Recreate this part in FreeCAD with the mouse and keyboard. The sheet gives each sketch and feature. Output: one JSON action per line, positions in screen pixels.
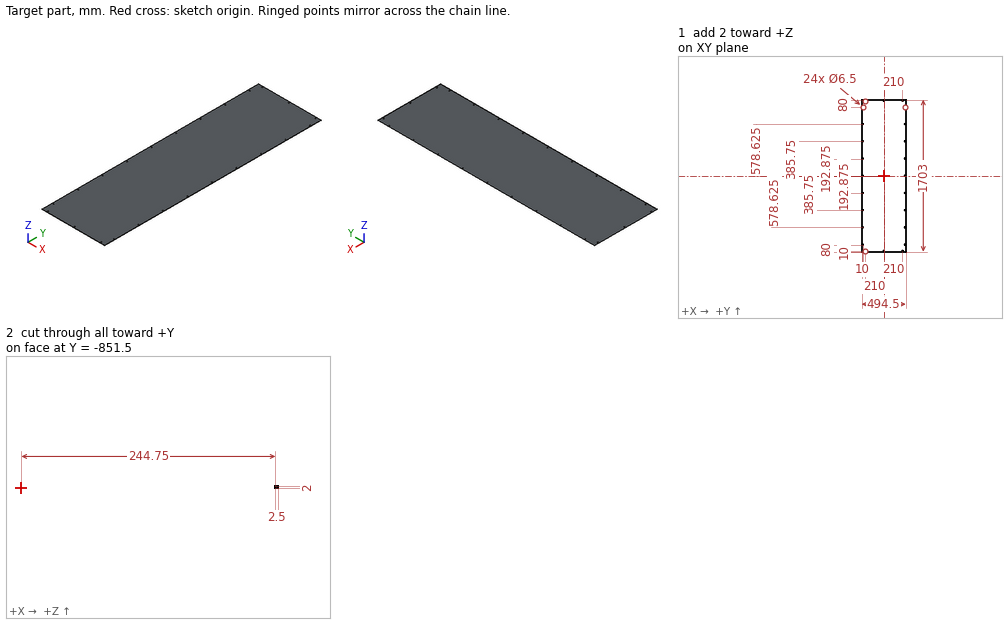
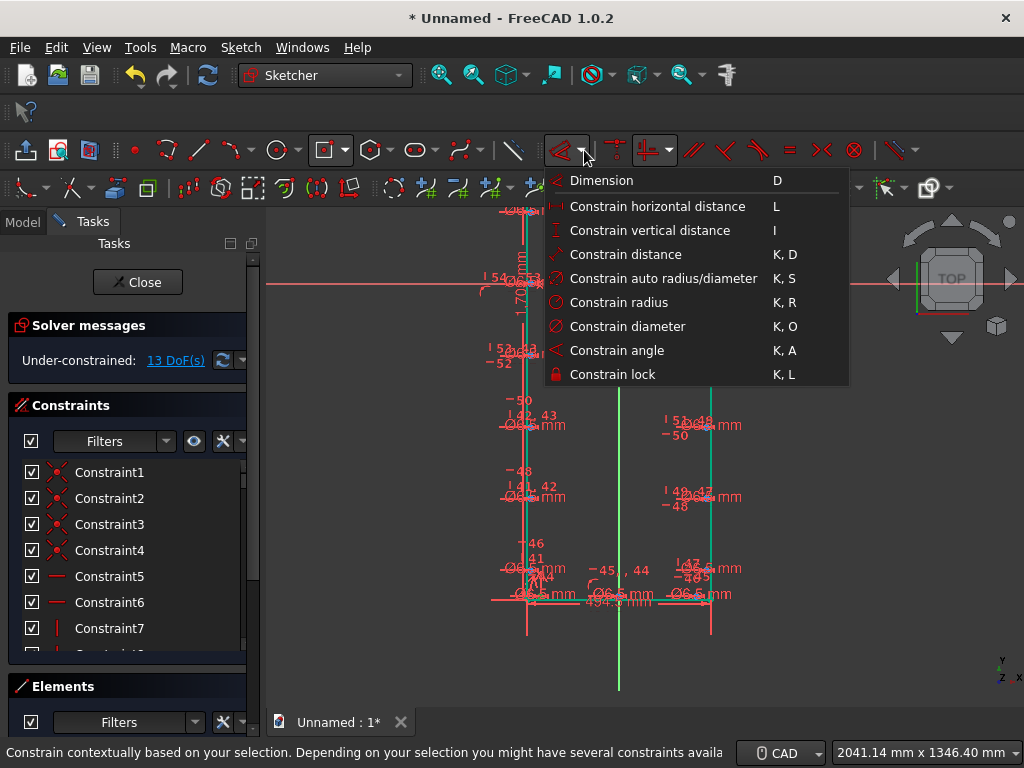
{"action": "left_click", "coordinate": [697, 206]}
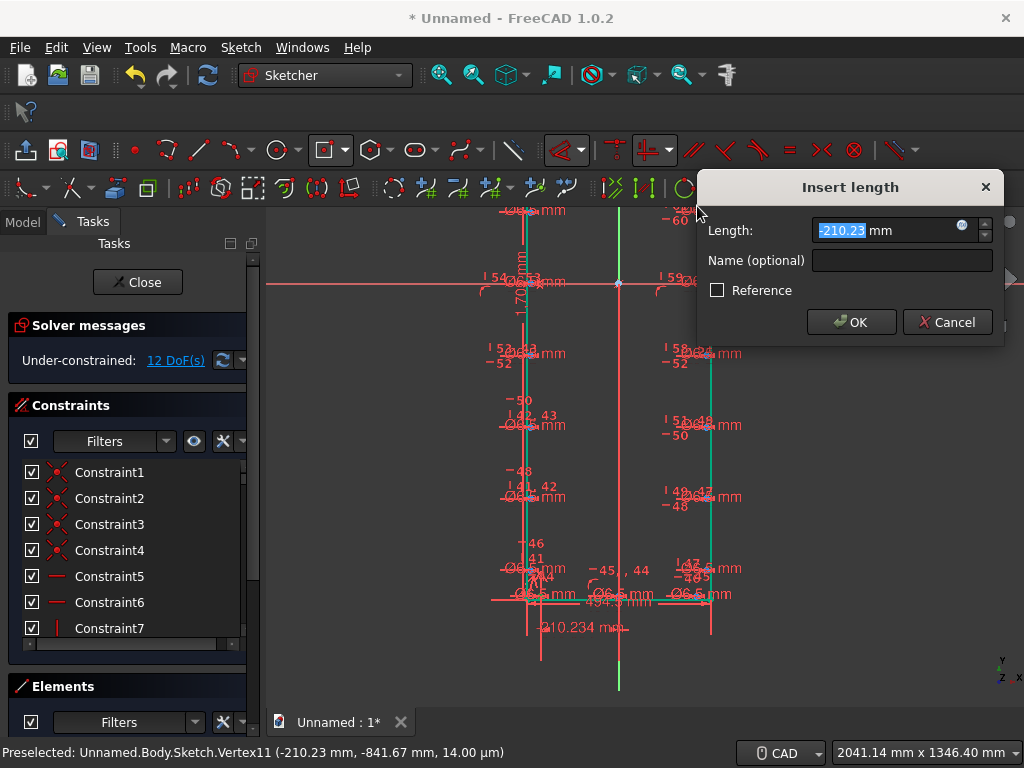
{"action": "type", "text": "-210"}
{"action": "key", "text": "Return"}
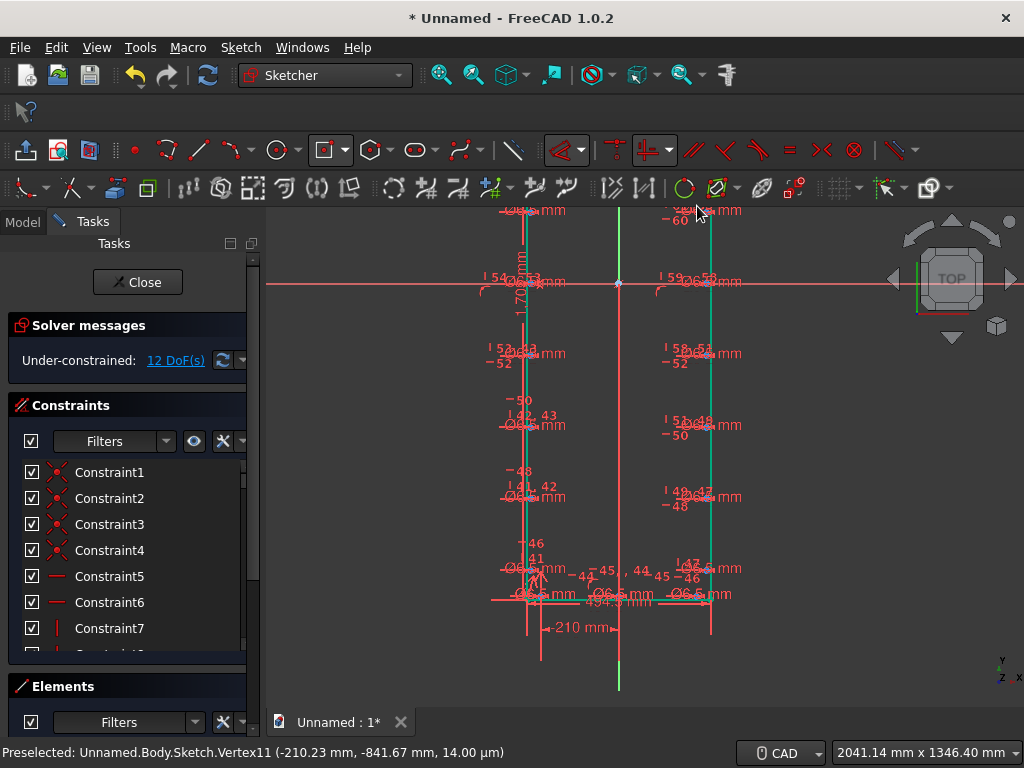
{"action": "left_click", "coordinate": [697, 596]}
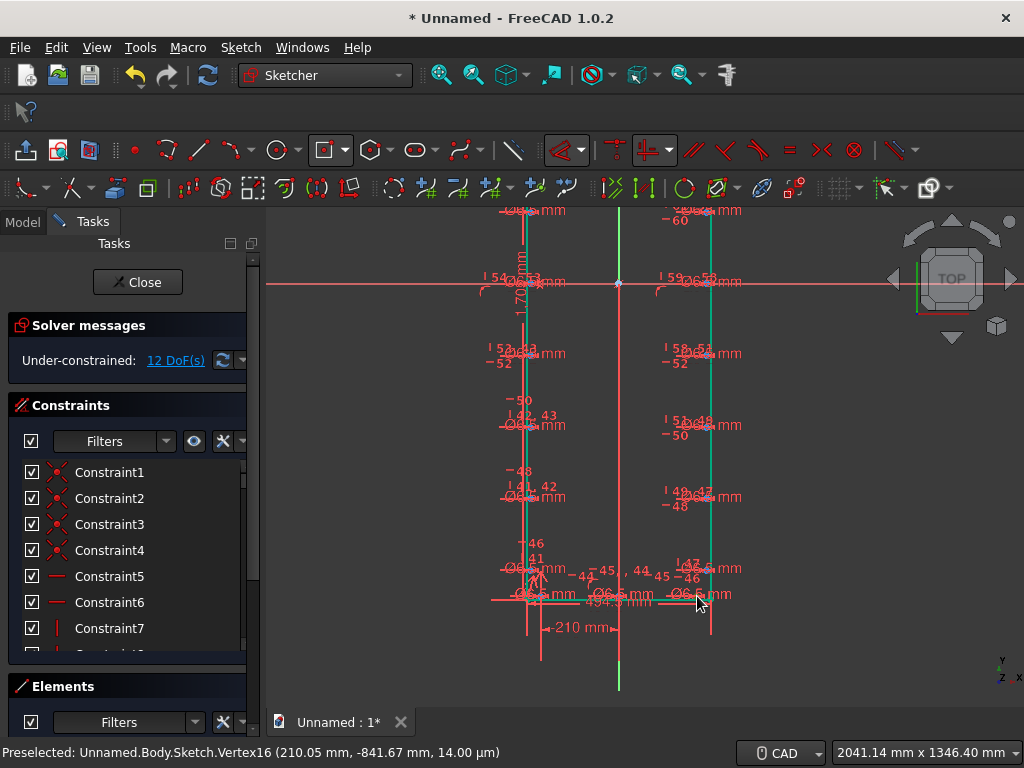
{"action": "left_click", "coordinate": [584, 150]}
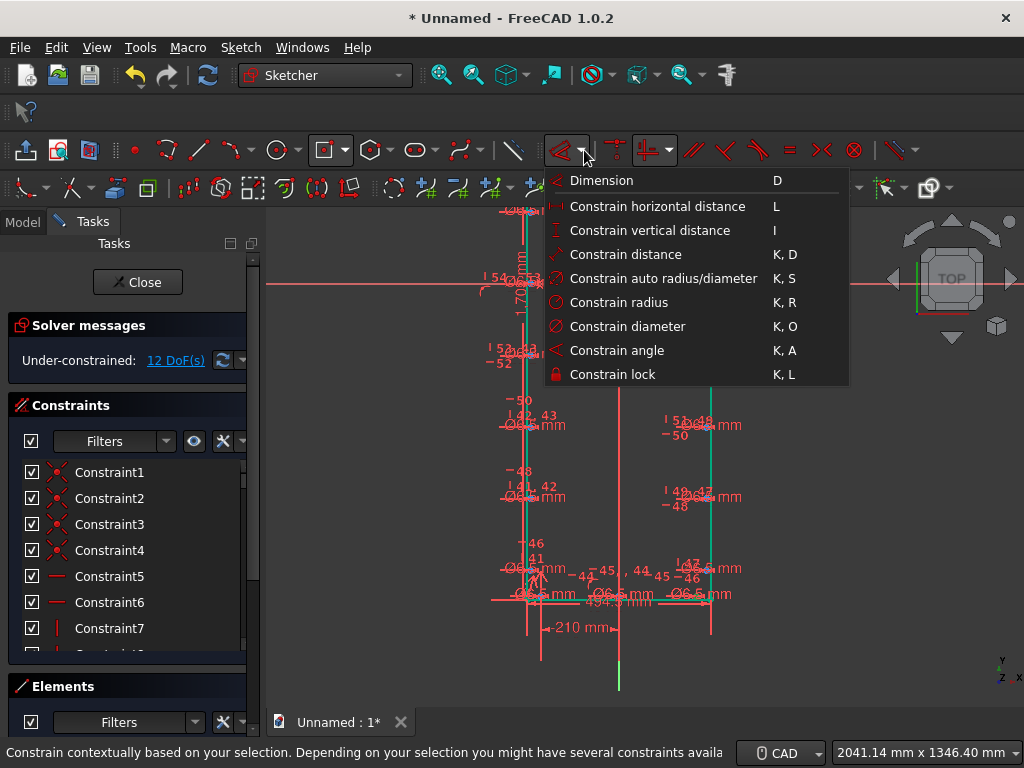
{"action": "left_click", "coordinate": [697, 206]}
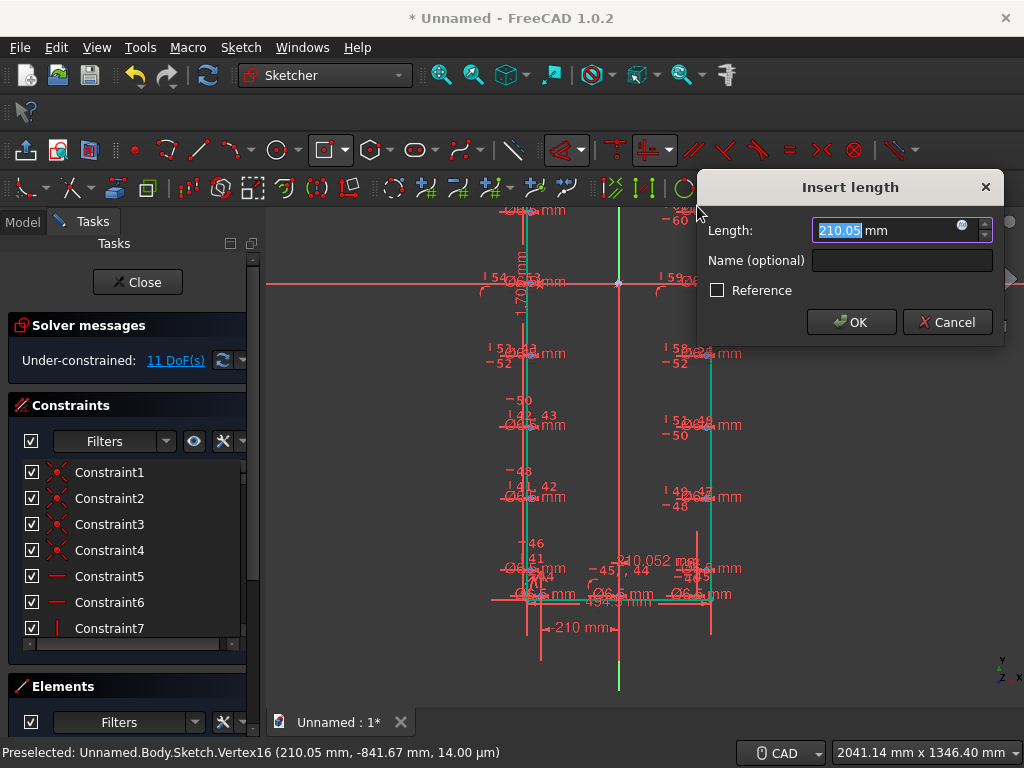
{"action": "type", "text": "210"}
{"action": "key", "text": "Return"}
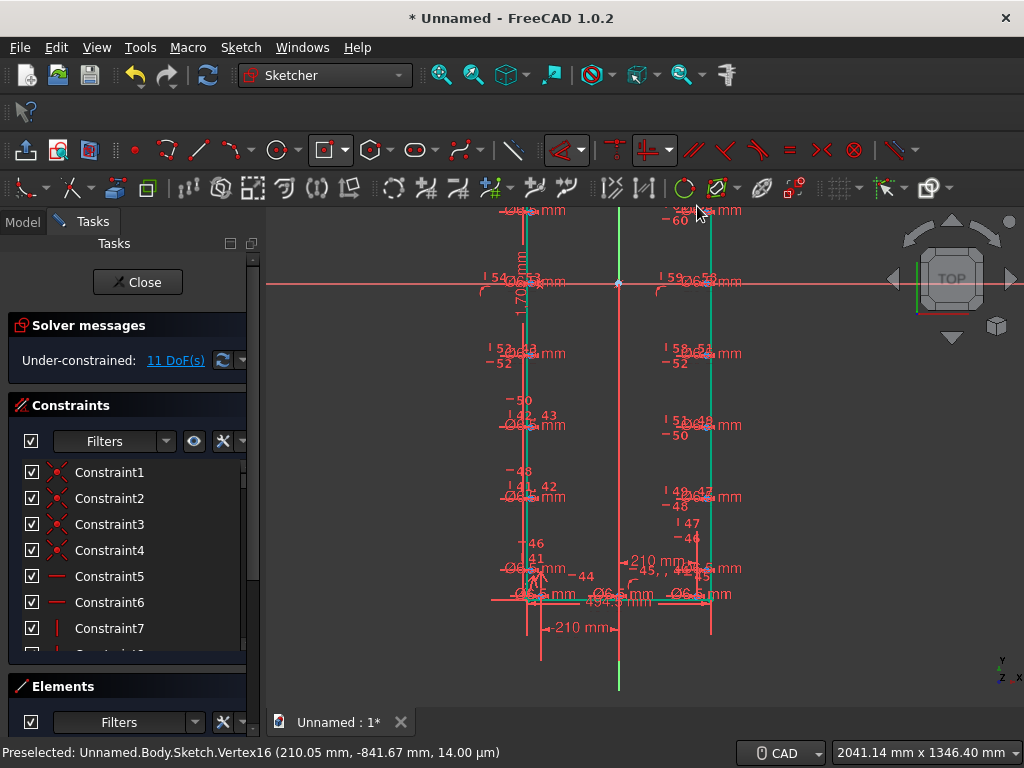
{"action": "scroll", "coordinate": [542, 598], "scroll_direction": "down", "scroll_amount": 4}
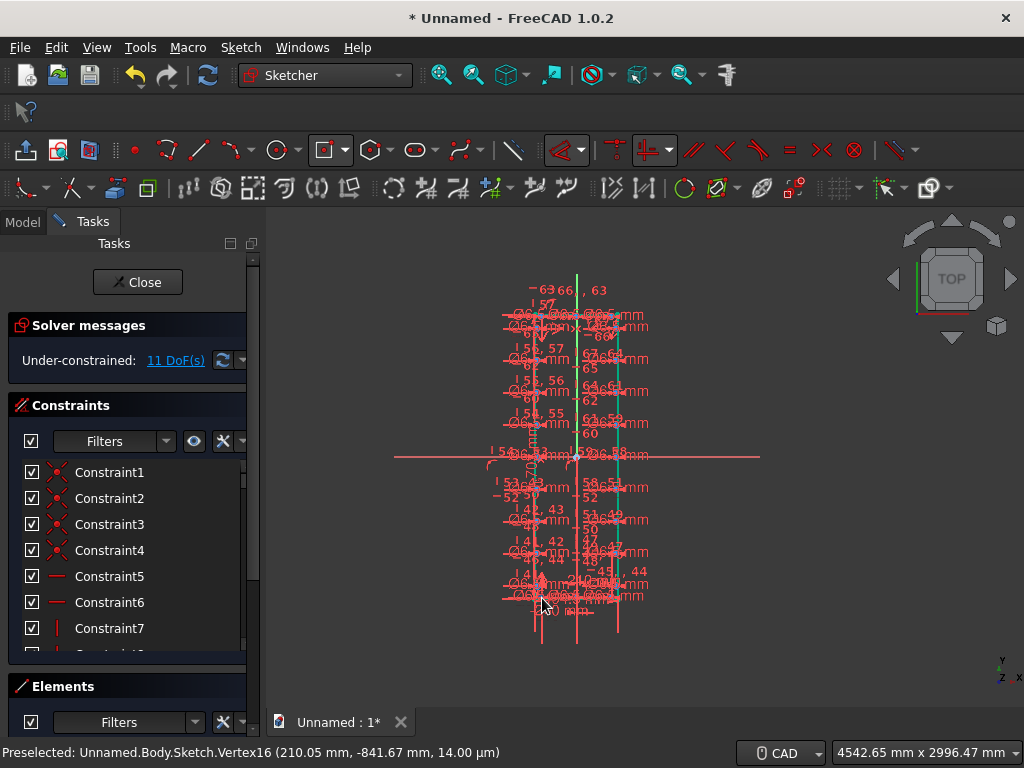
{"action": "scroll", "coordinate": [612, 317], "scroll_direction": "up", "scroll_amount": 4}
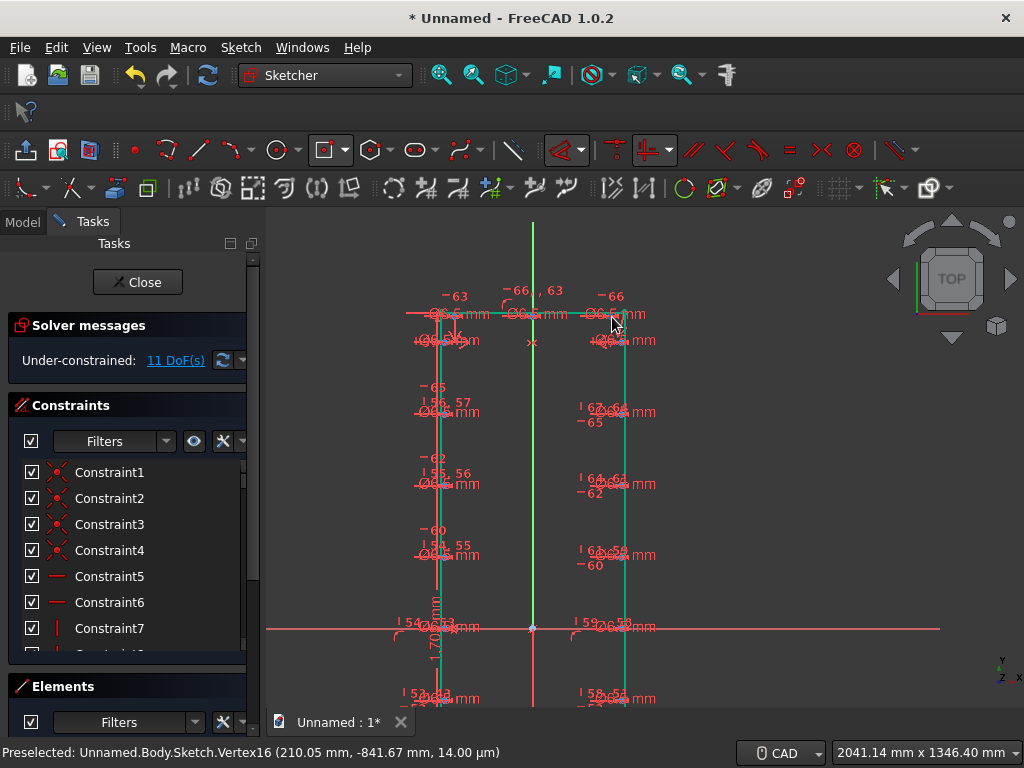
{"action": "left_click", "coordinate": [611, 316]}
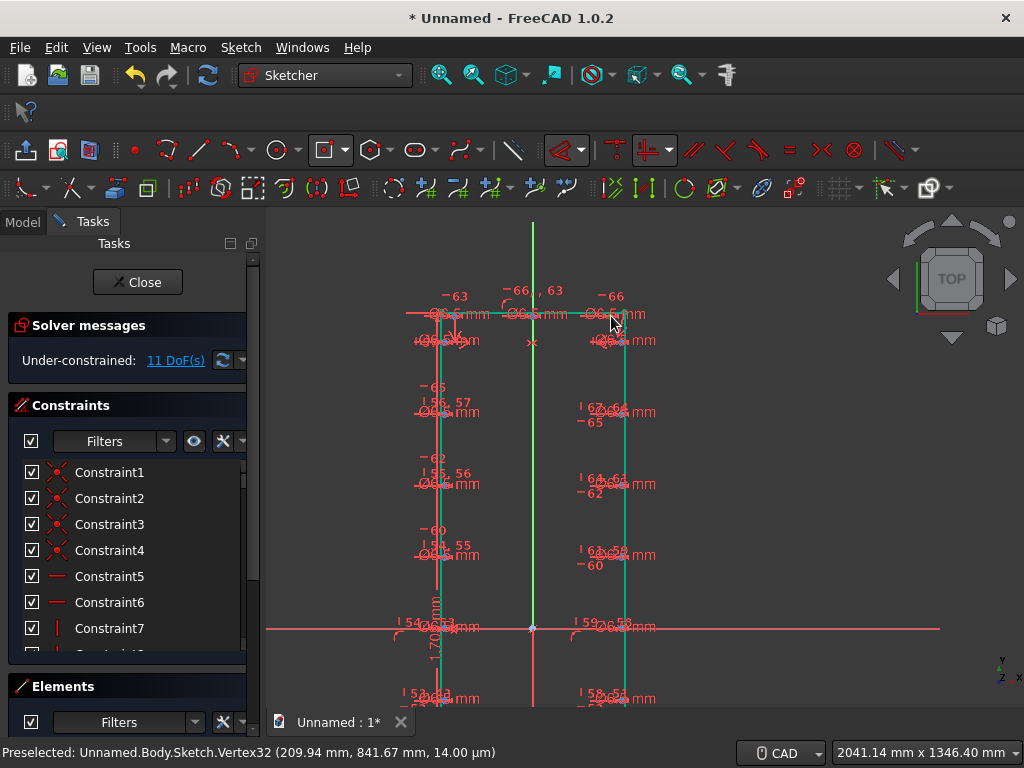
{"action": "left_click", "coordinate": [584, 150]}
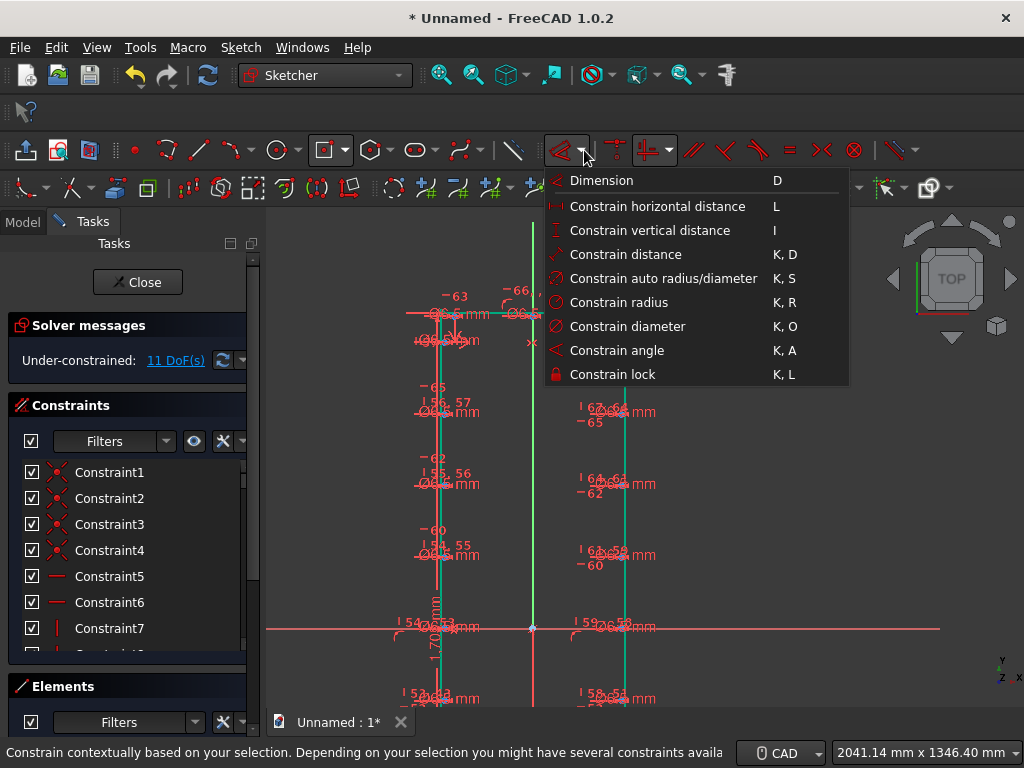
{"action": "left_click", "coordinate": [697, 206]}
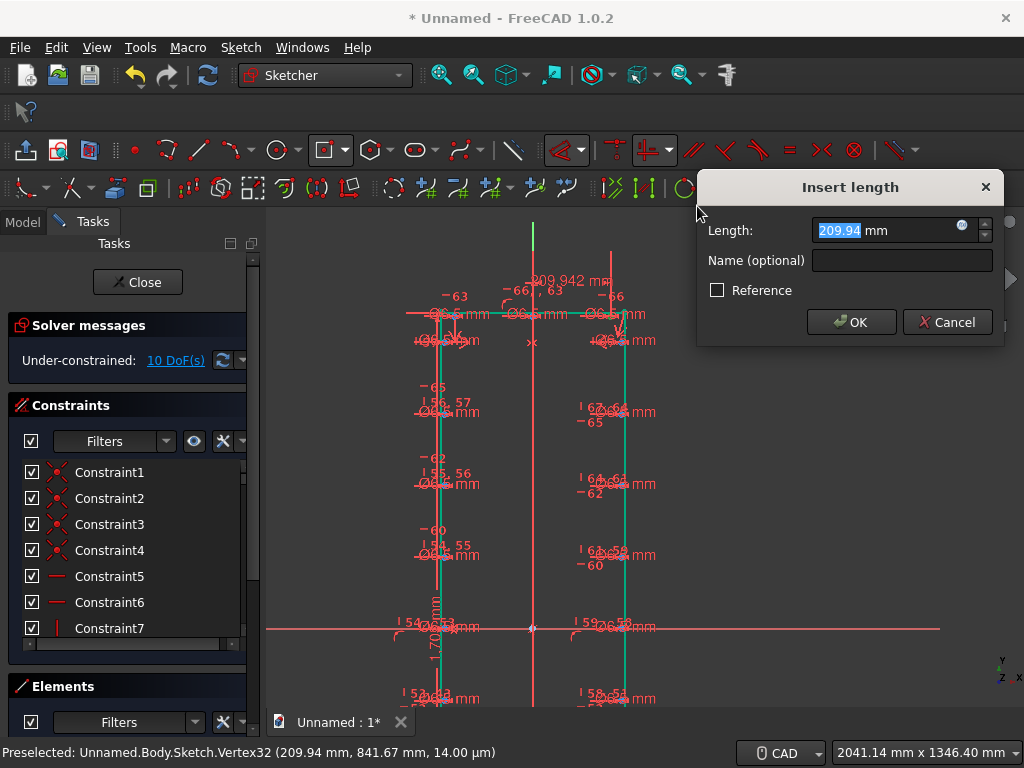
{"action": "type", "text": "210"}
{"action": "key", "text": "Return"}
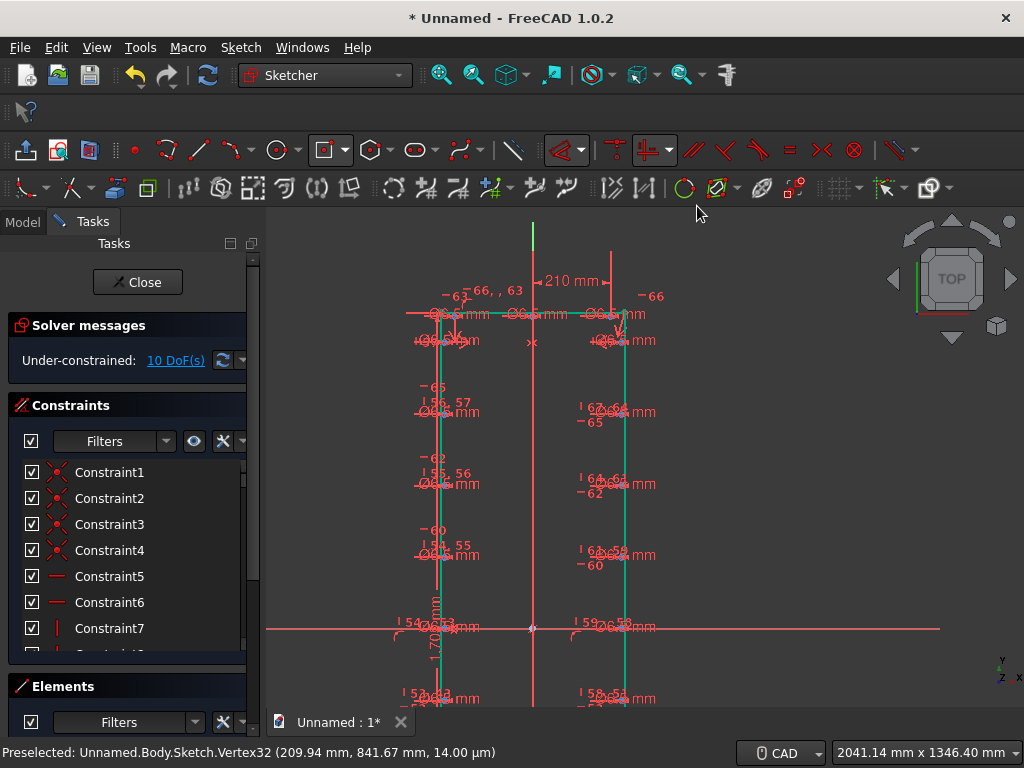
{"action": "scroll", "coordinate": [612, 317], "scroll_direction": "down", "scroll_amount": 4}